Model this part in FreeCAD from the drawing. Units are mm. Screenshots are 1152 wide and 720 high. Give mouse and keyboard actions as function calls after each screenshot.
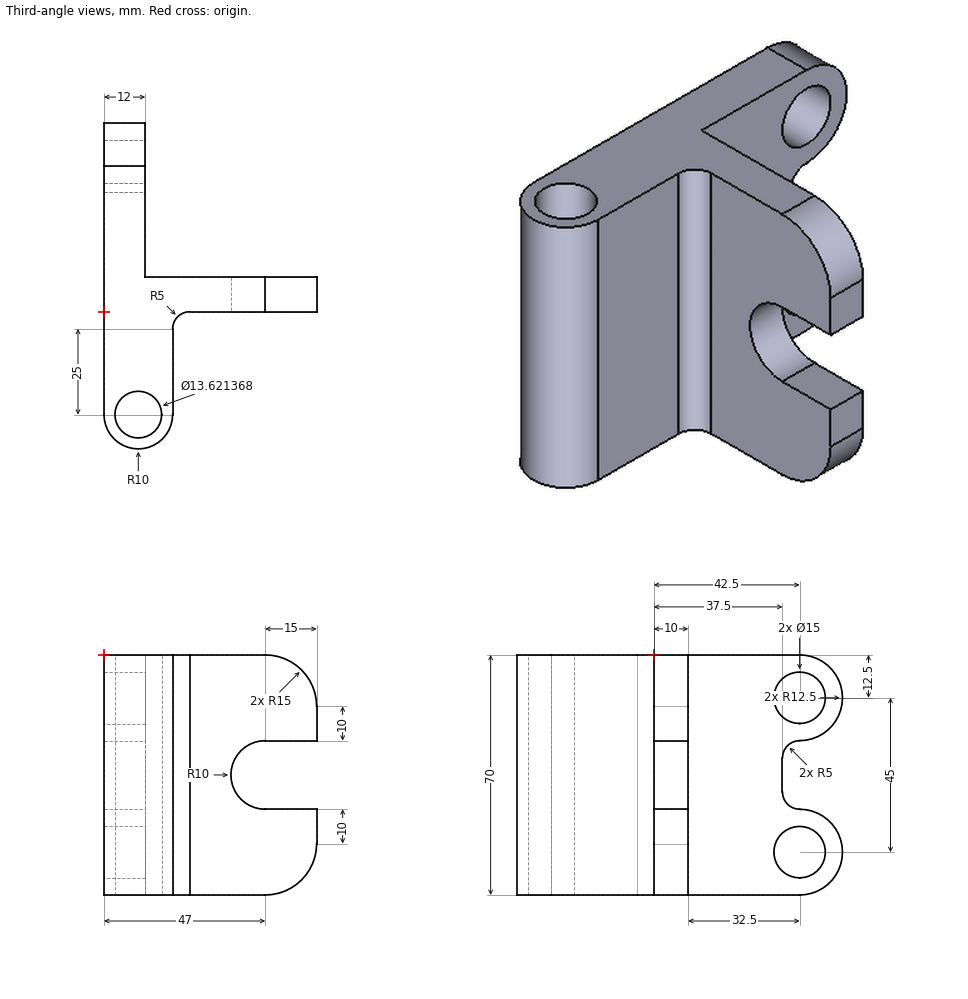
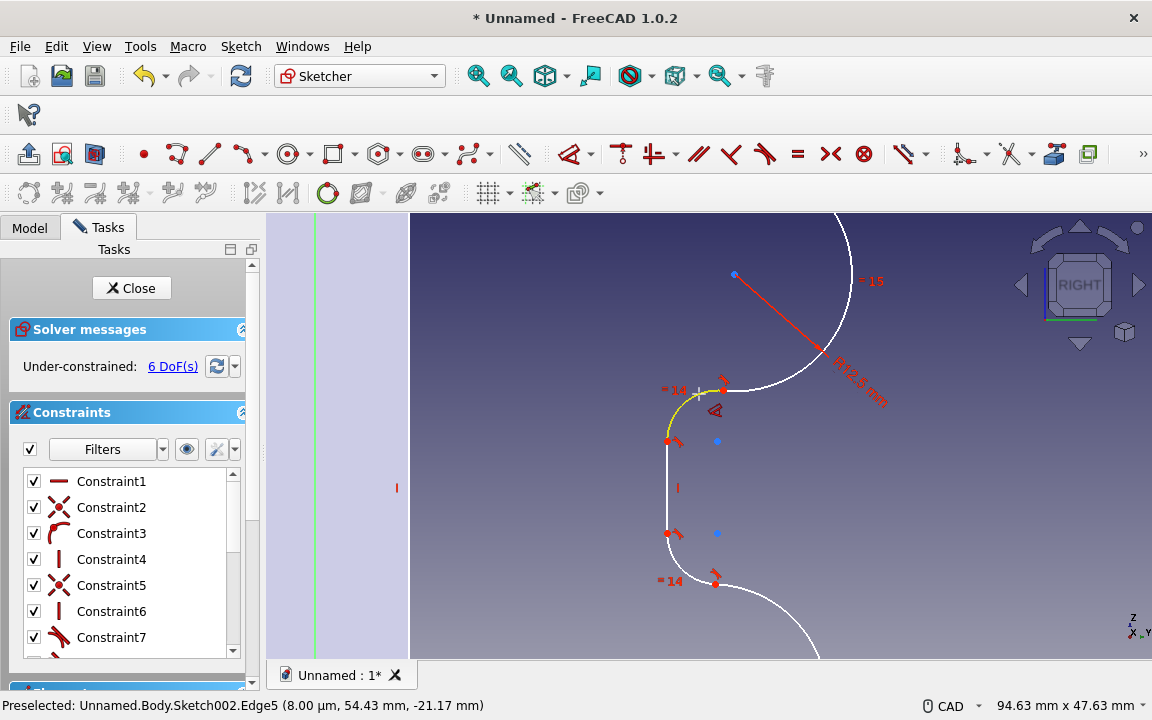
click(698, 395)
click(685, 366)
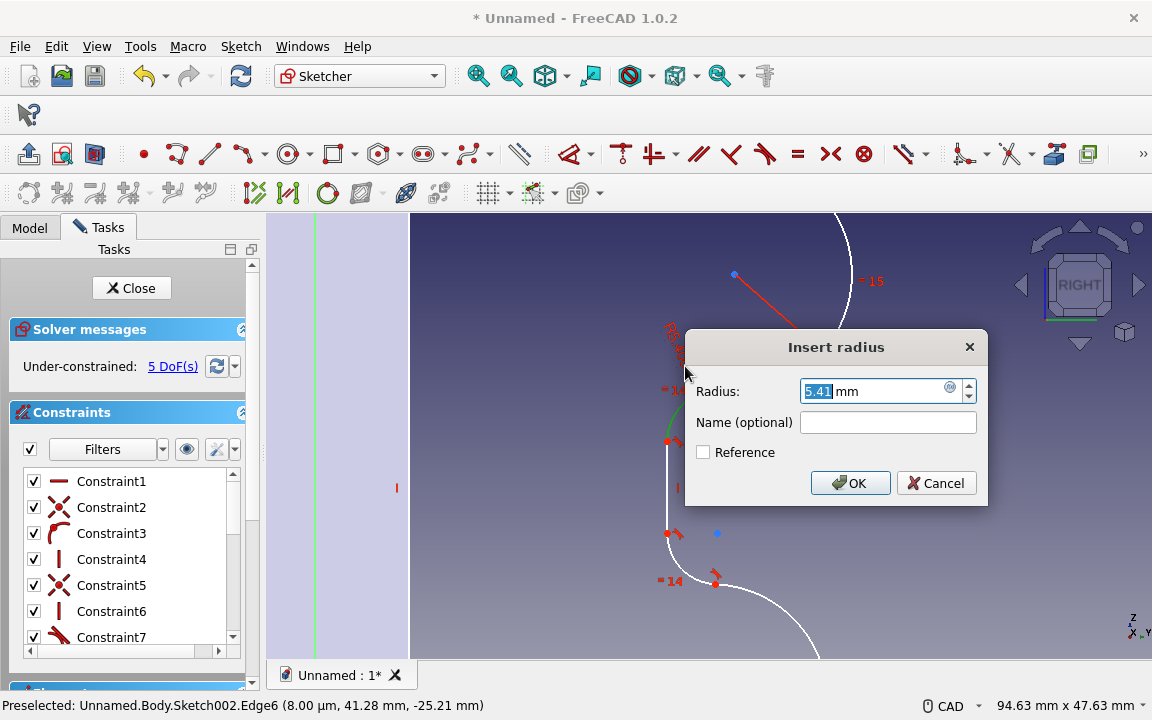
text(5)
key(Return)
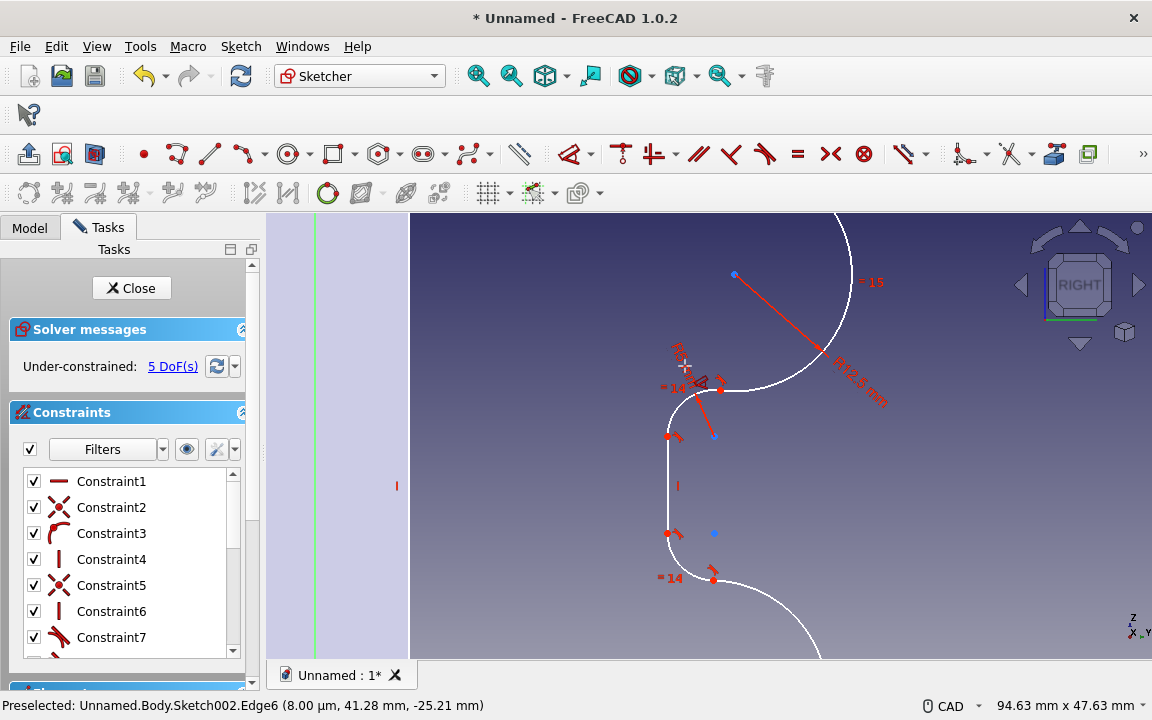
click(409, 617)
click(375, 436)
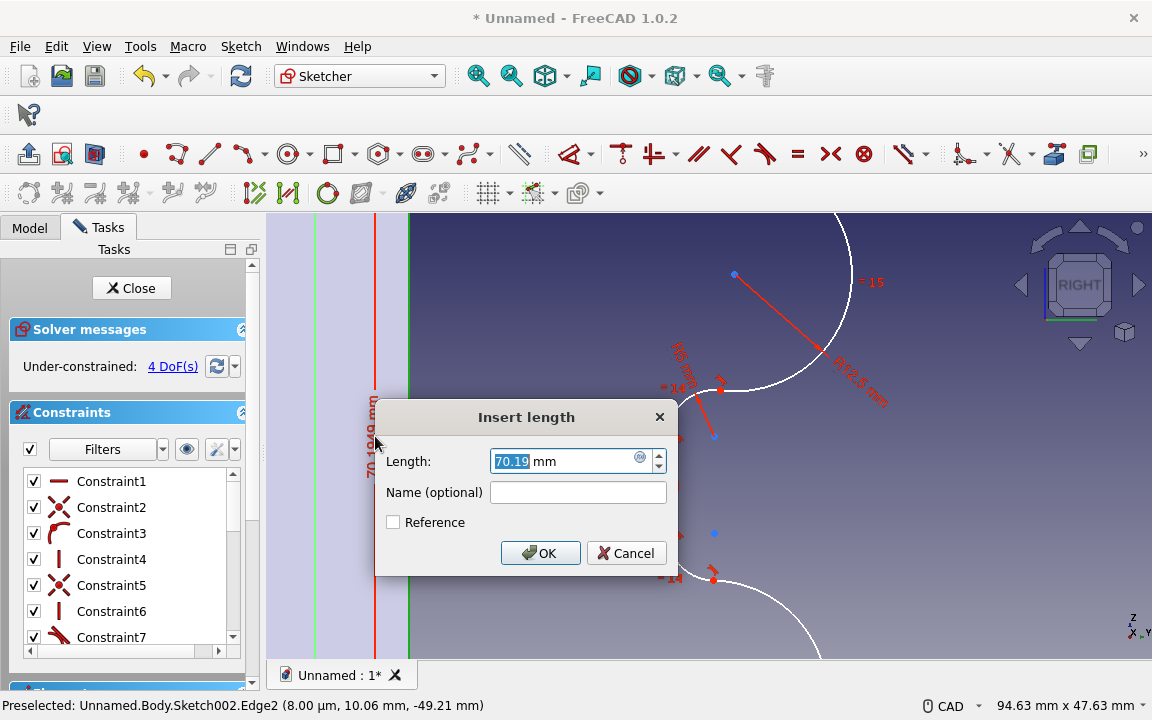
text(70)
key(Return)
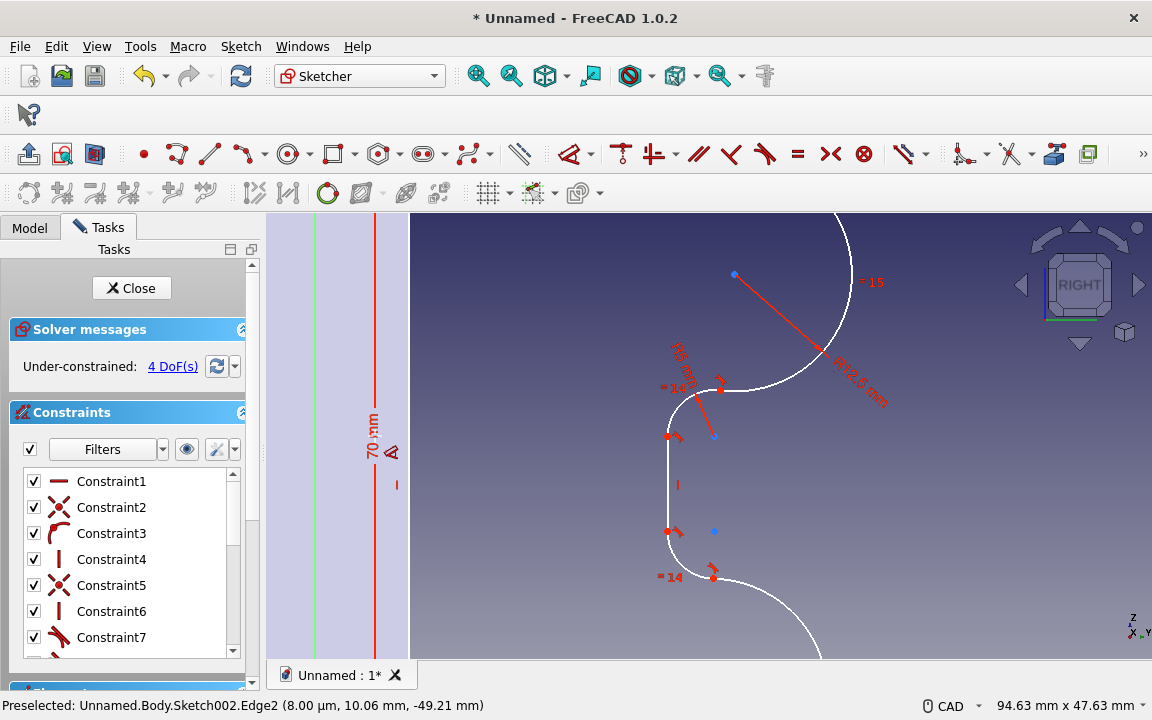
scroll(696, 396, down, 4)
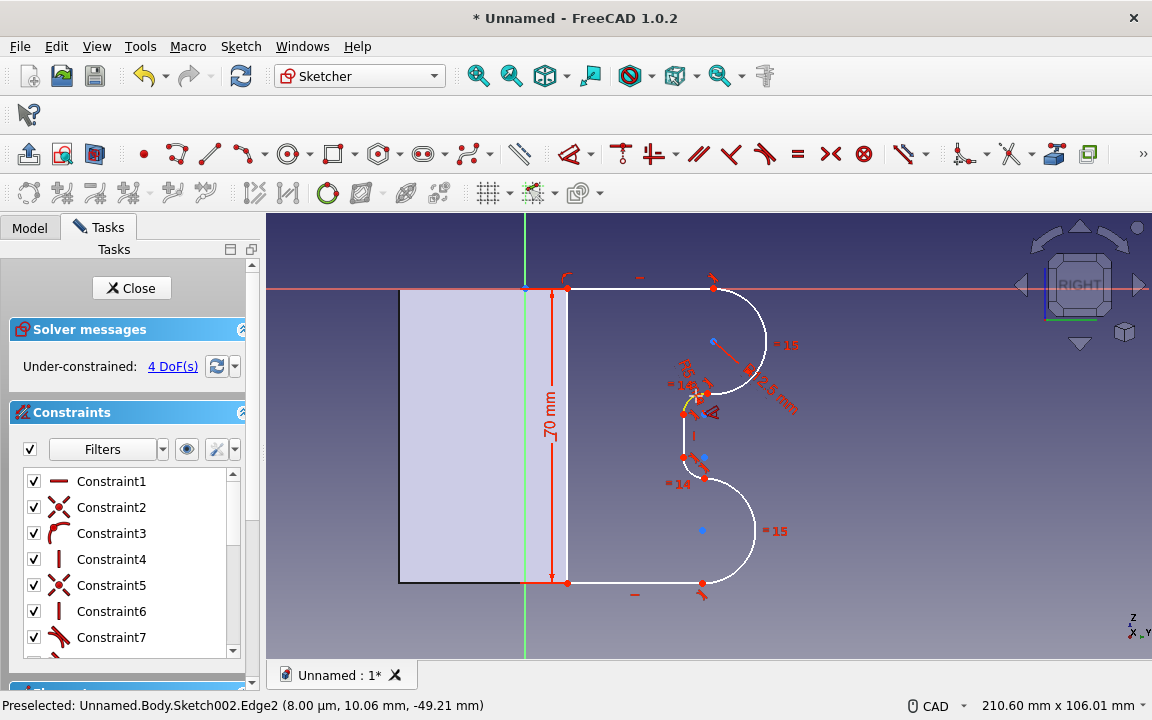
click(567, 583)
click(546, 255)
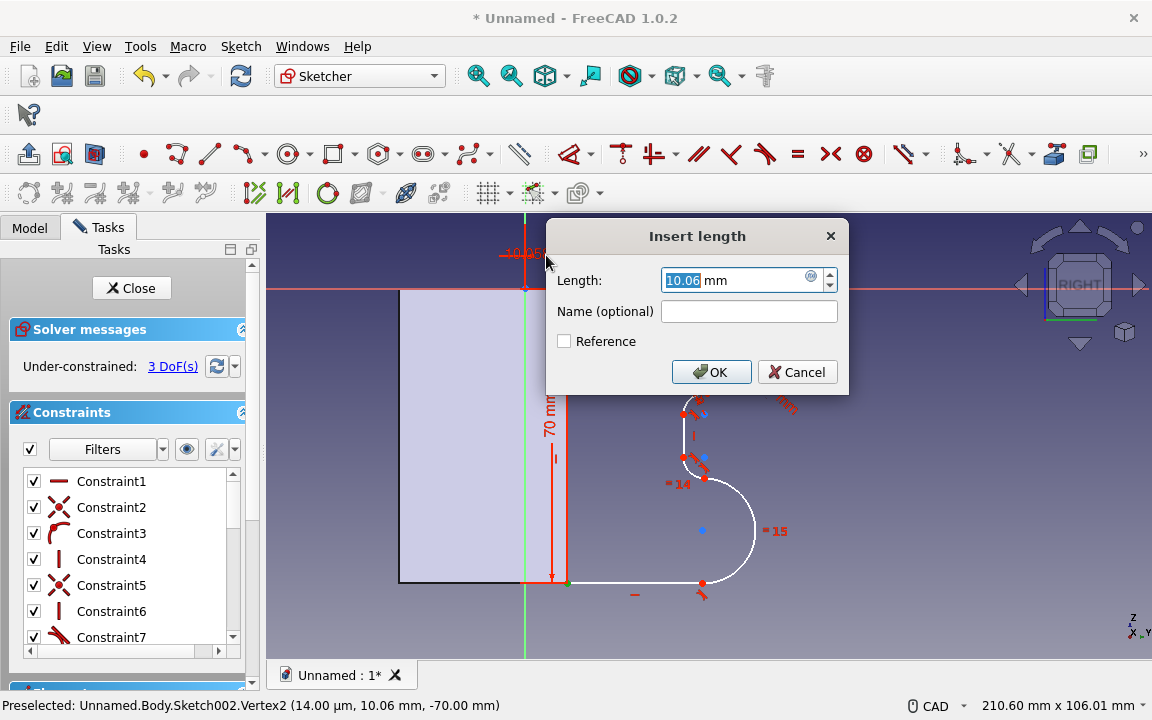
text(10)
key(Return)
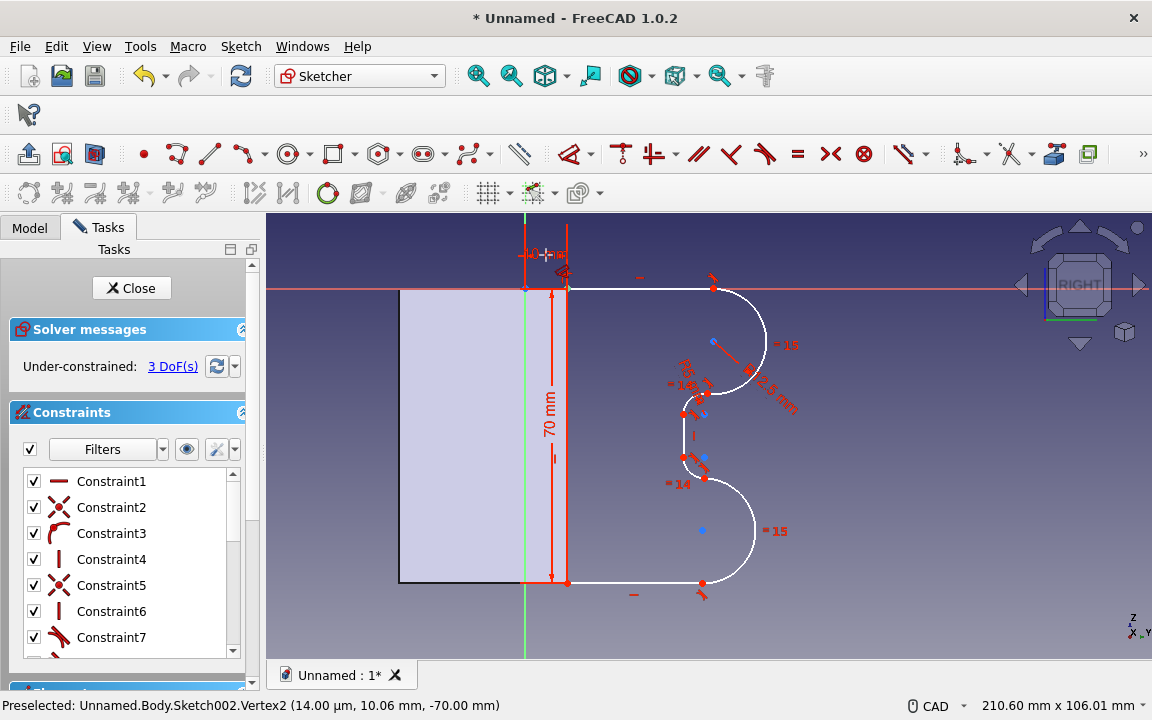
click(662, 583)
click(635, 617)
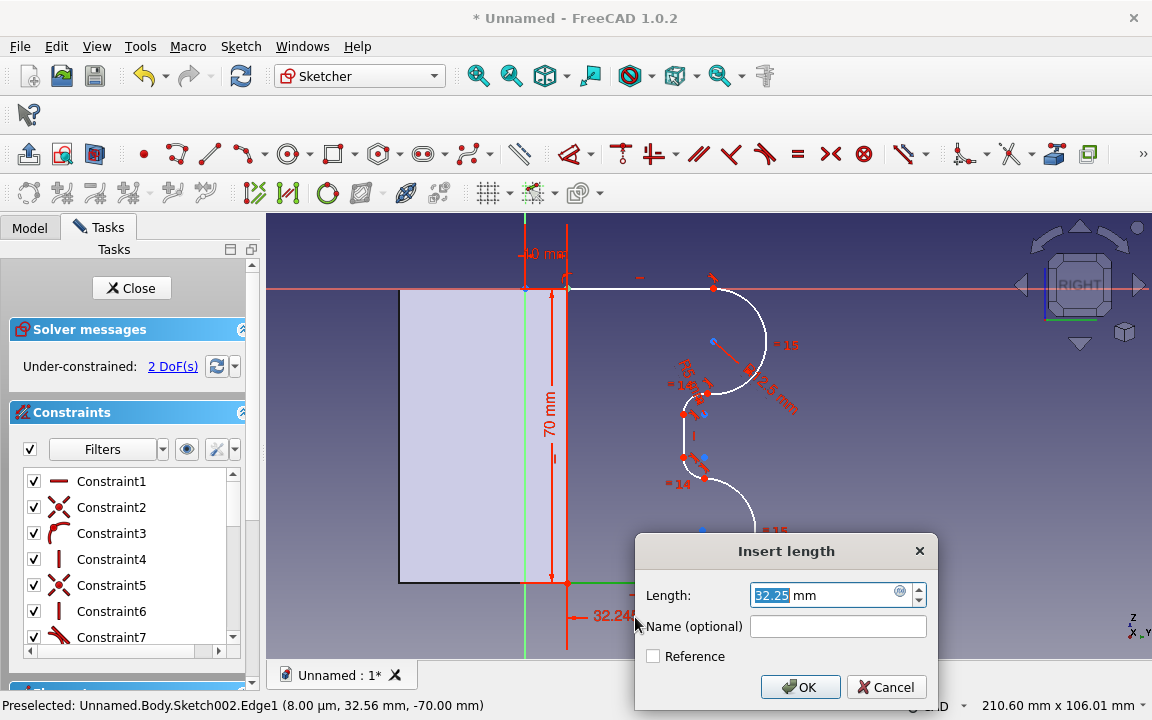
text(32.5)
key(Return)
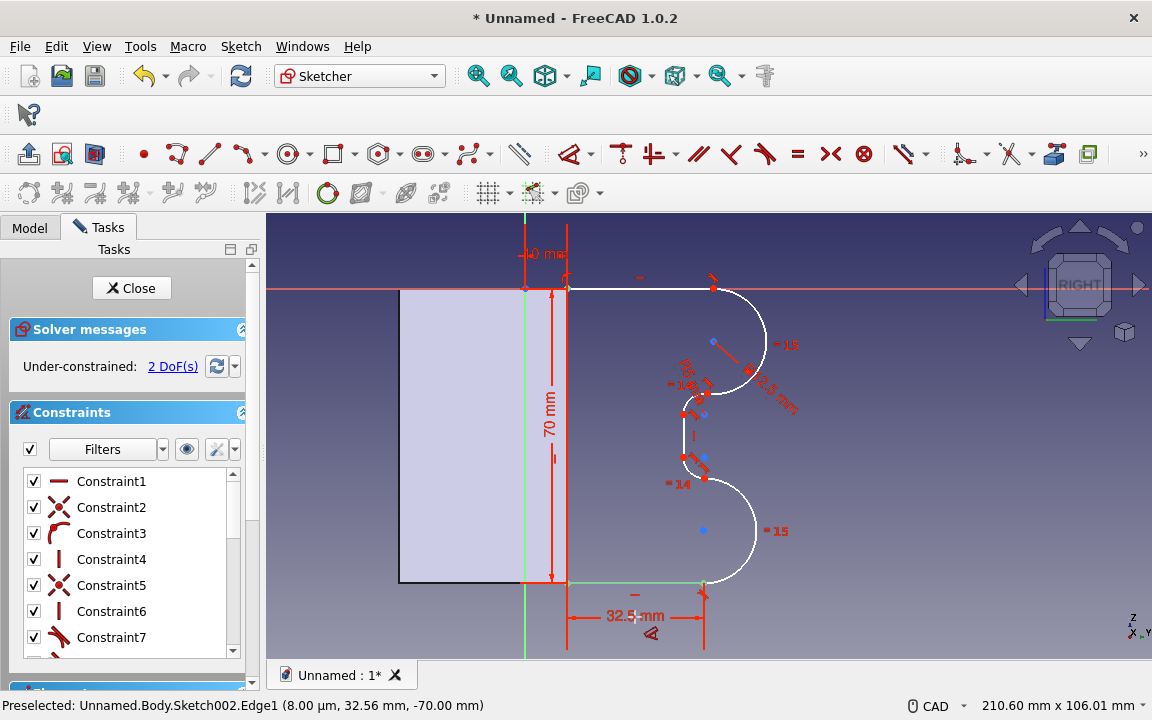
click(611, 289)
click(640, 255)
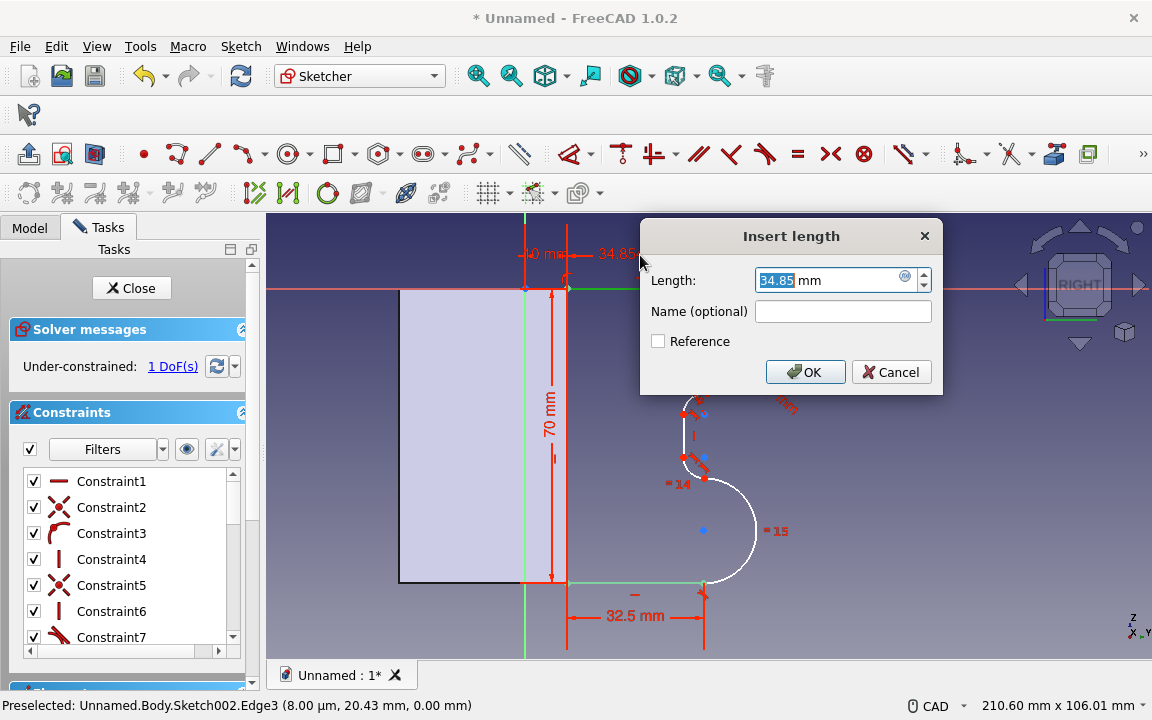
text(32.5)
key(Return)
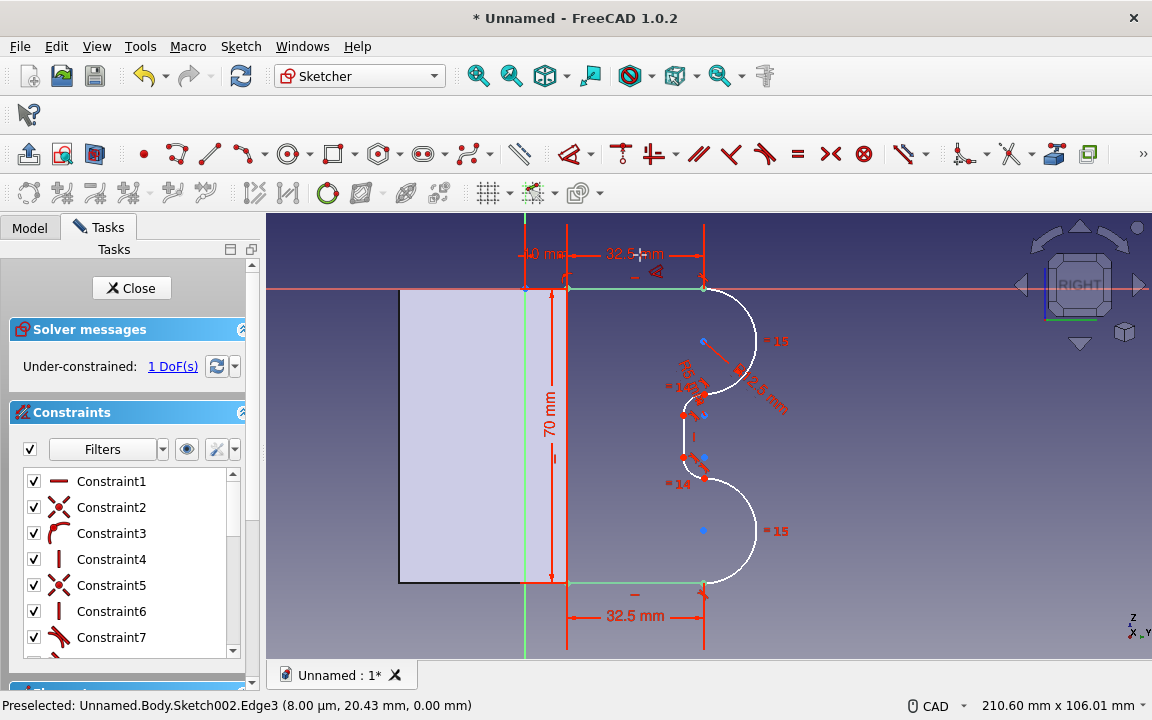
click(684, 415)
click(604, 449)